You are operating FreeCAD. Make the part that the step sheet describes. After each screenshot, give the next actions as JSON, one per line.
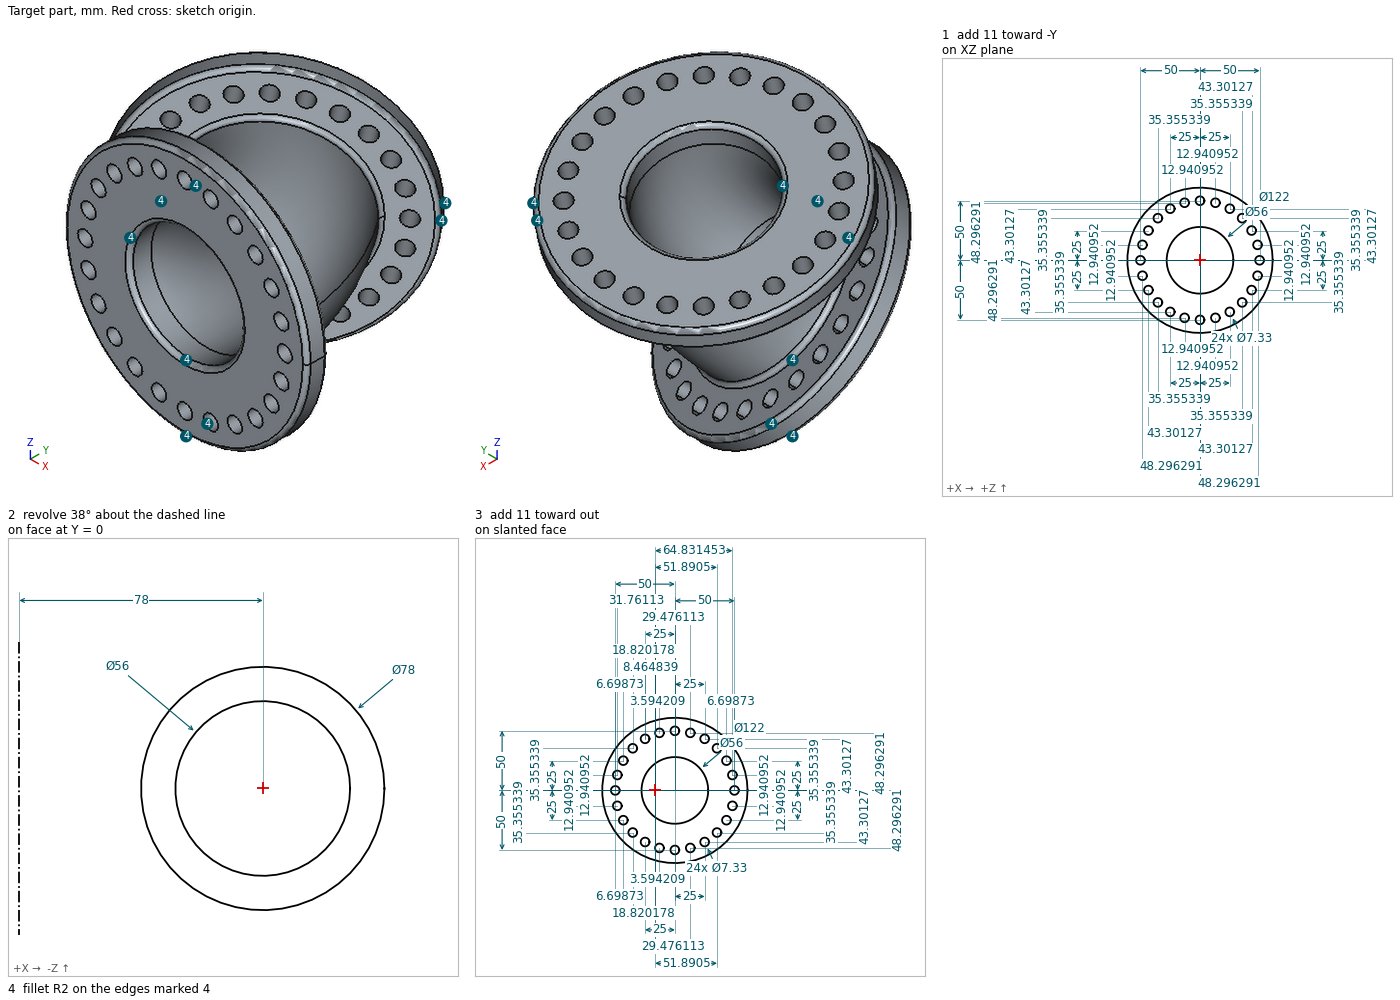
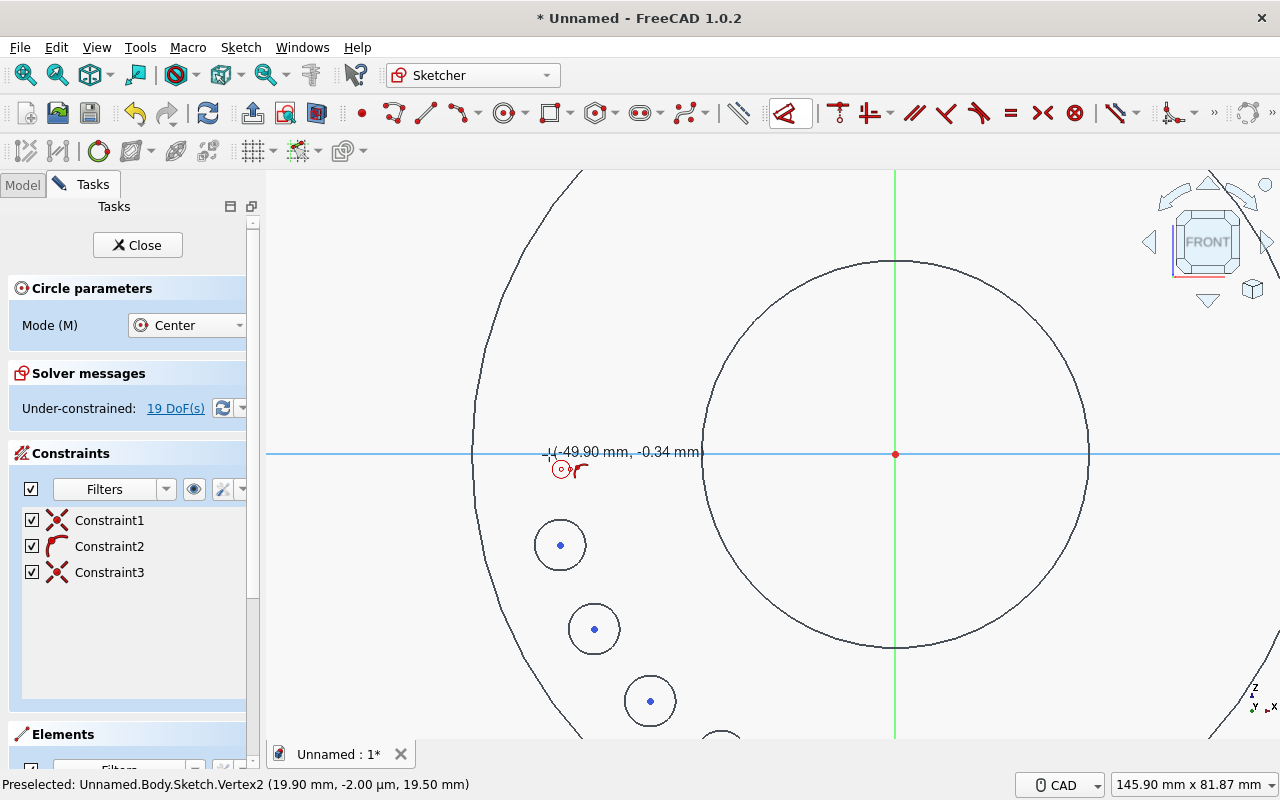
{"action": "left_click", "coordinate": [548, 454]}
{"action": "left_click", "coordinate": [566, 436]}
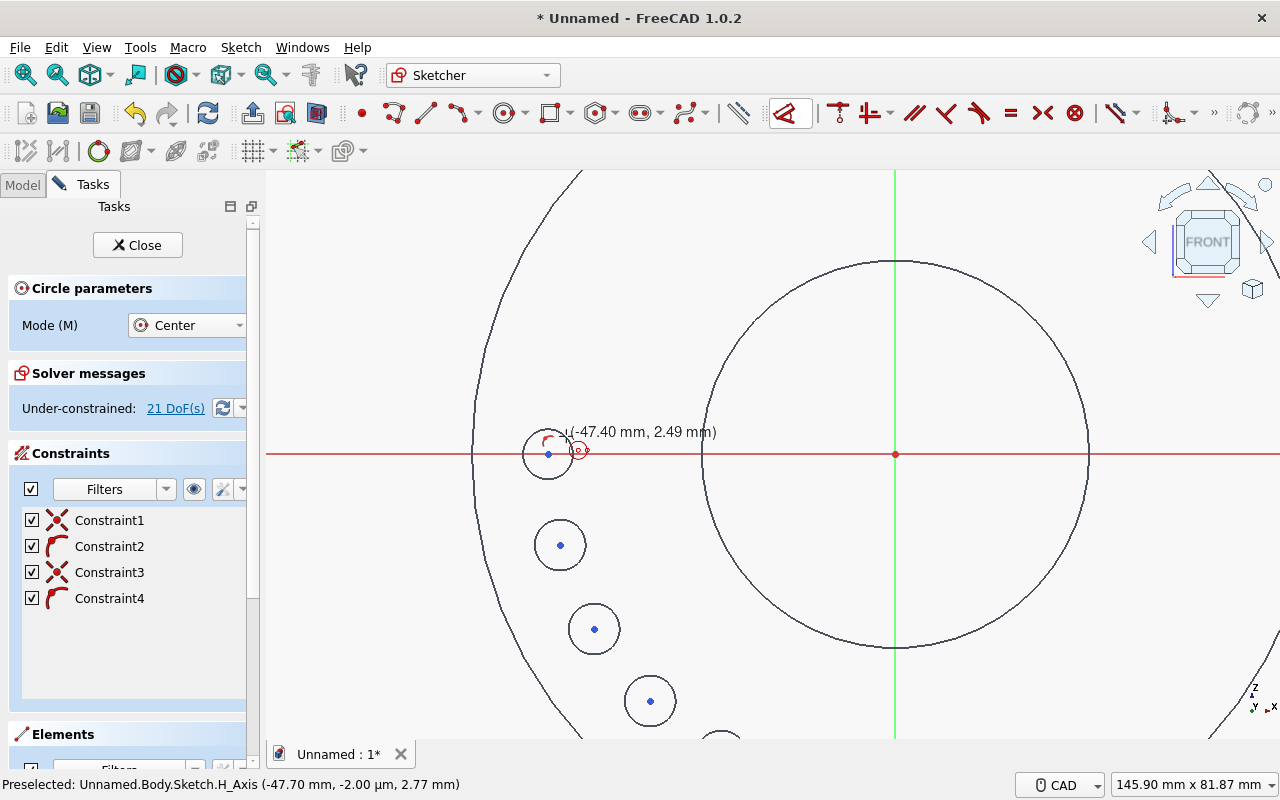
{"action": "left_click", "coordinate": [560, 364]}
{"action": "left_click", "coordinate": [578, 346]}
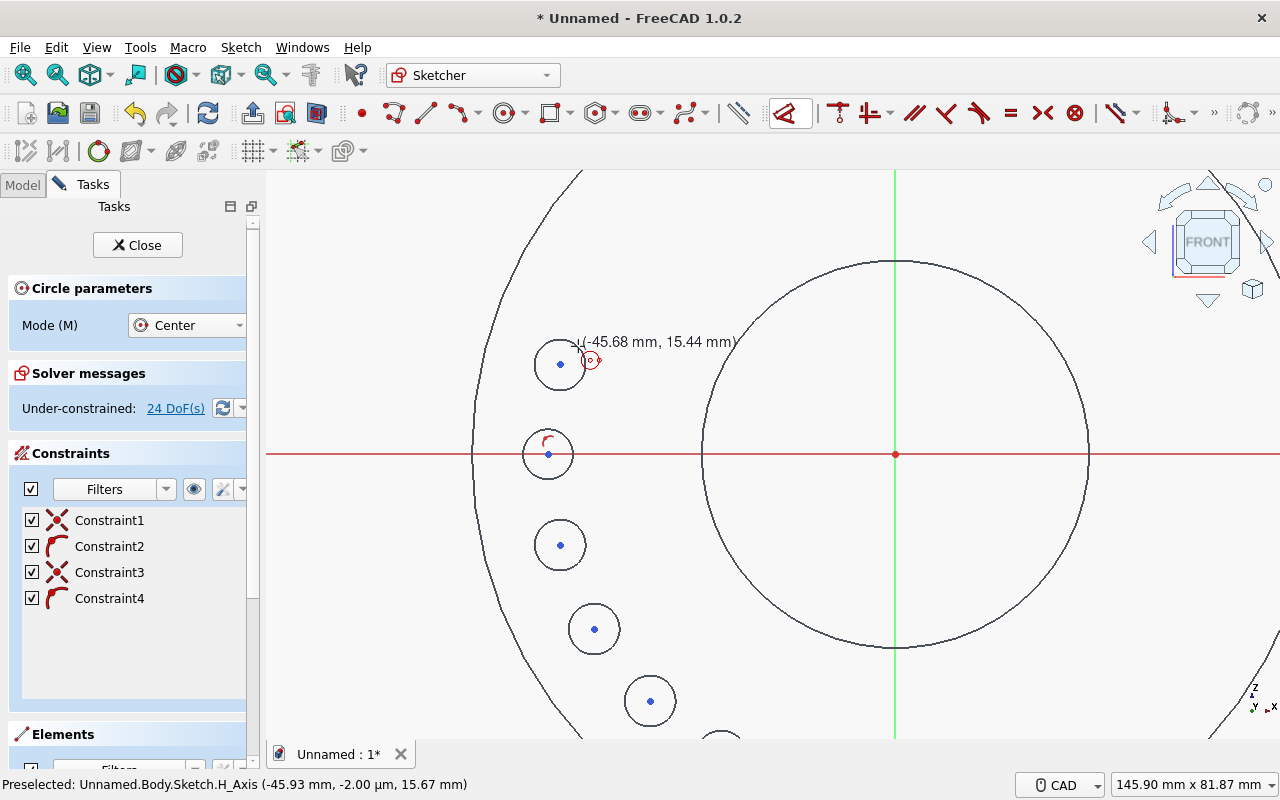
{"action": "left_click", "coordinate": [595, 281]}
{"action": "left_click", "coordinate": [613, 263]}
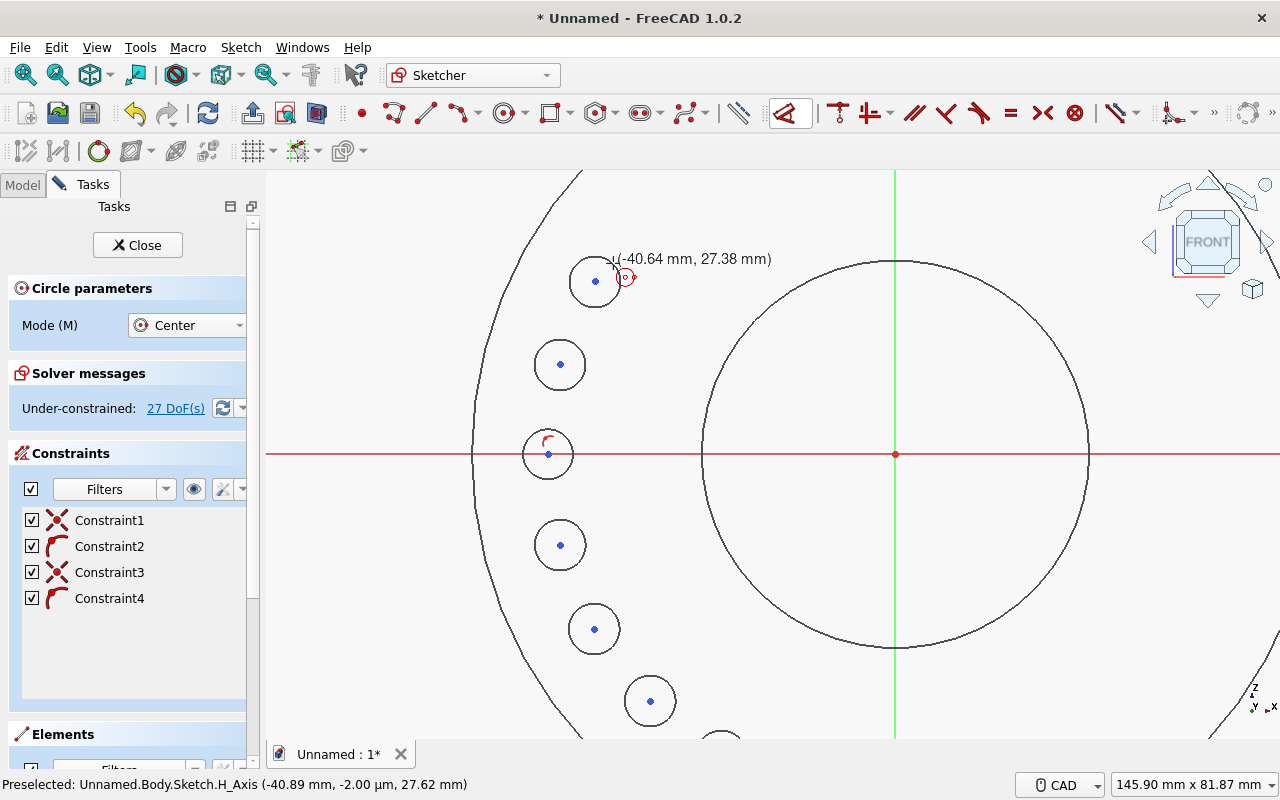
{"action": "left_click", "coordinate": [650, 209]}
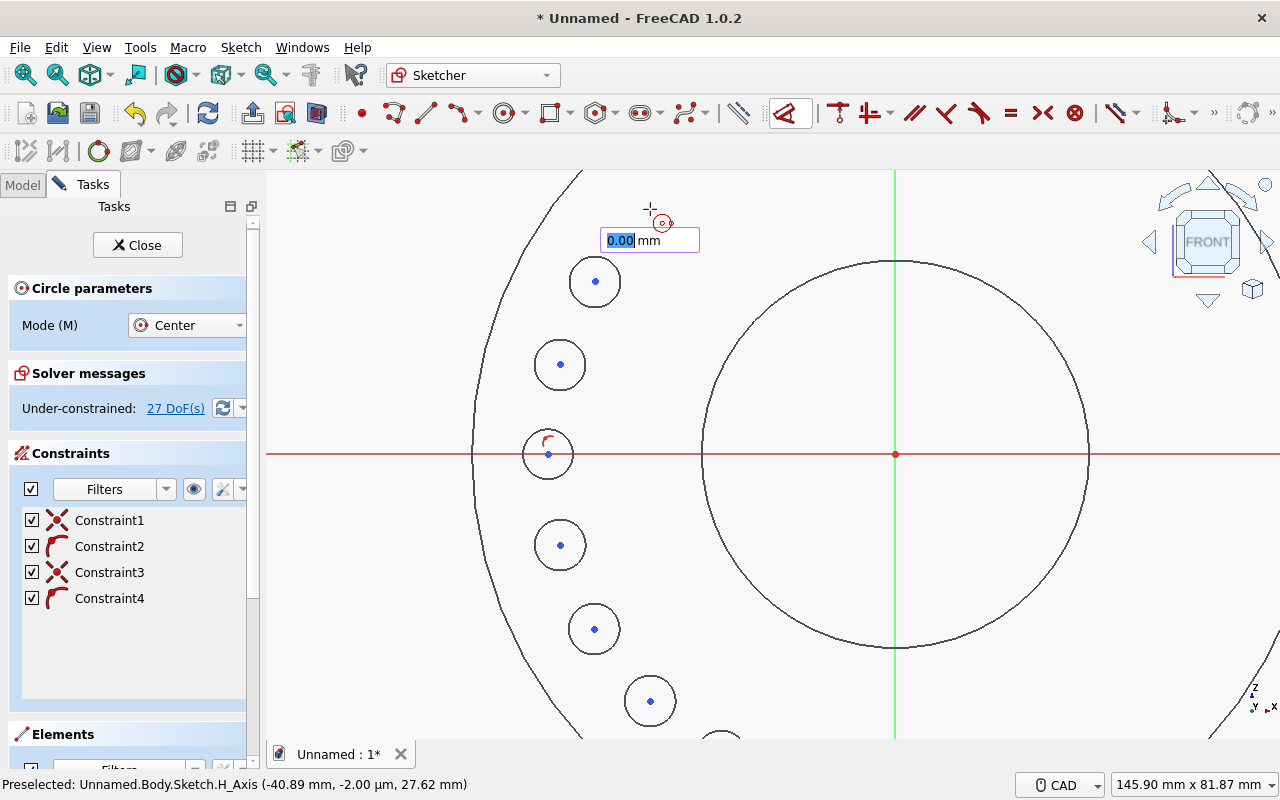
{"action": "scroll", "coordinate": [549, 455], "scroll_direction": "down", "scroll_amount": 4}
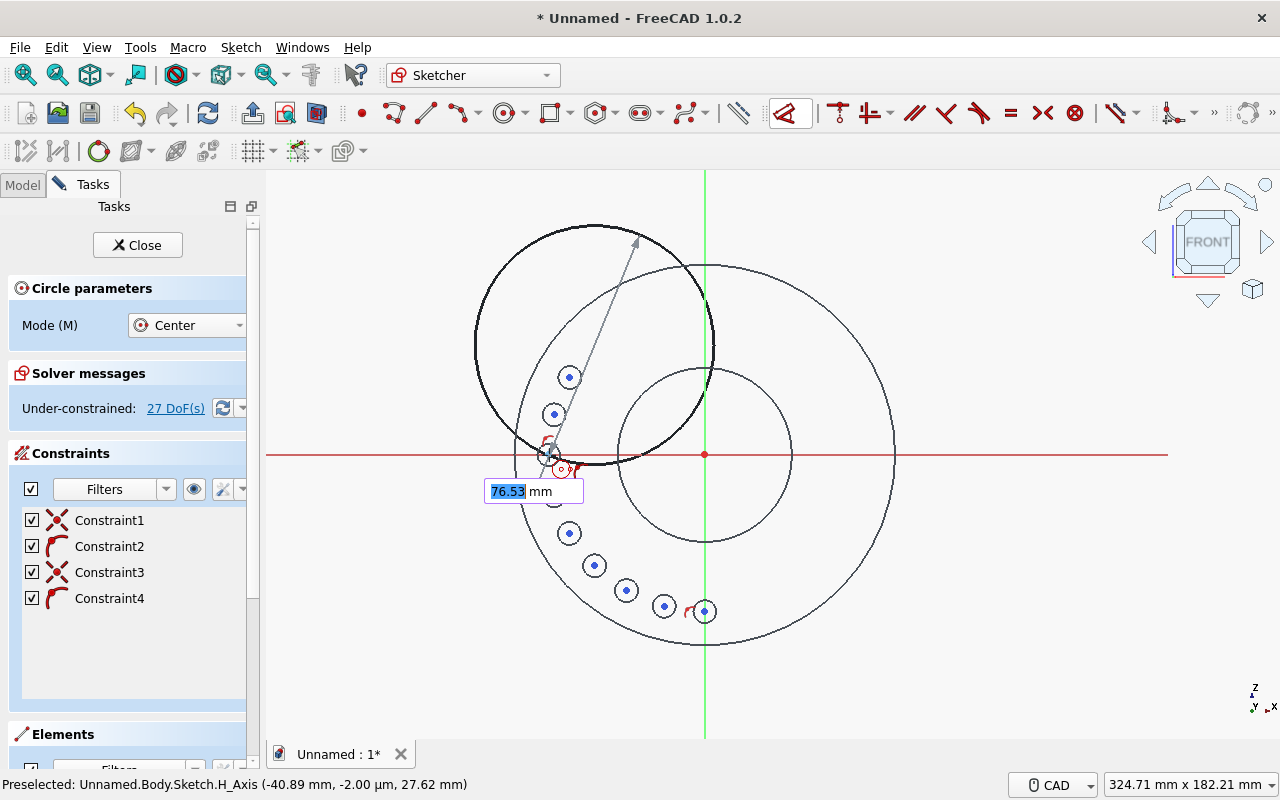
{"action": "scroll", "coordinate": [603, 336], "scroll_direction": "up", "scroll_amount": 2}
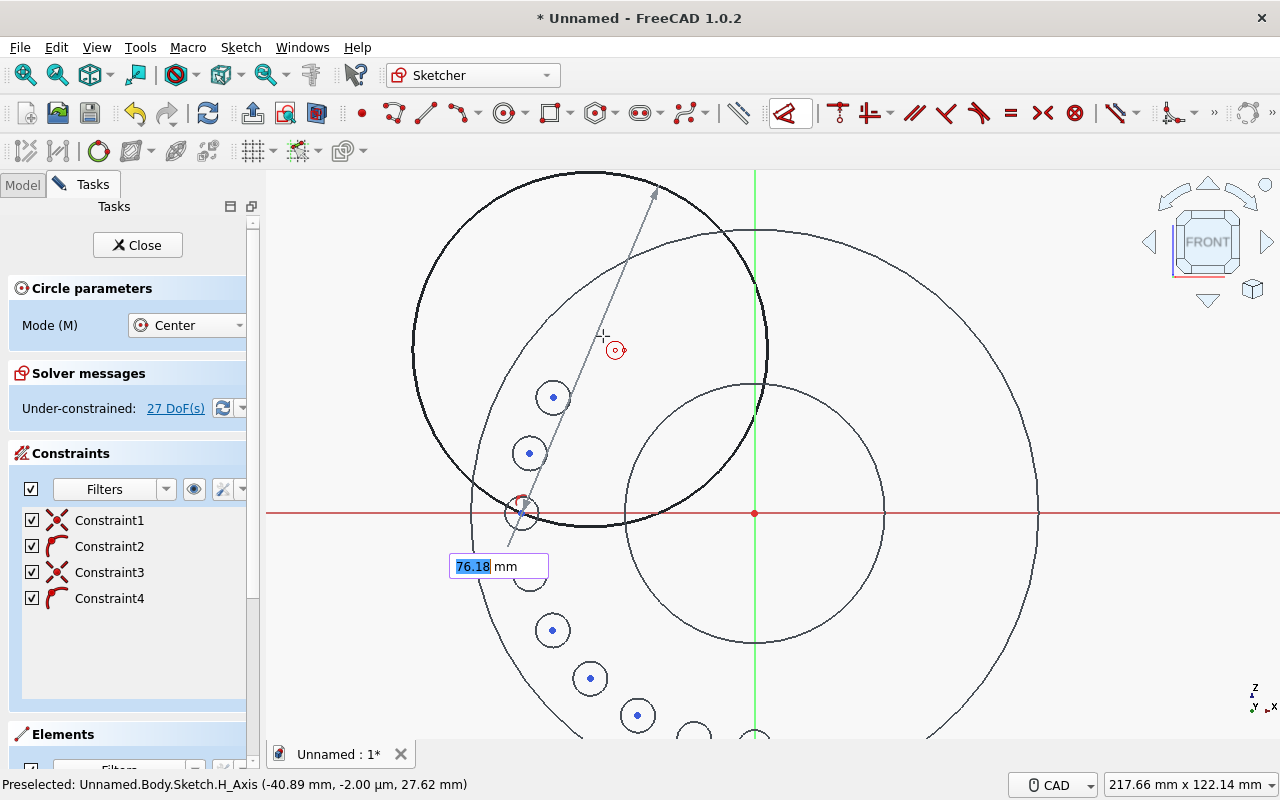
{"action": "left_click", "coordinate": [602, 337]}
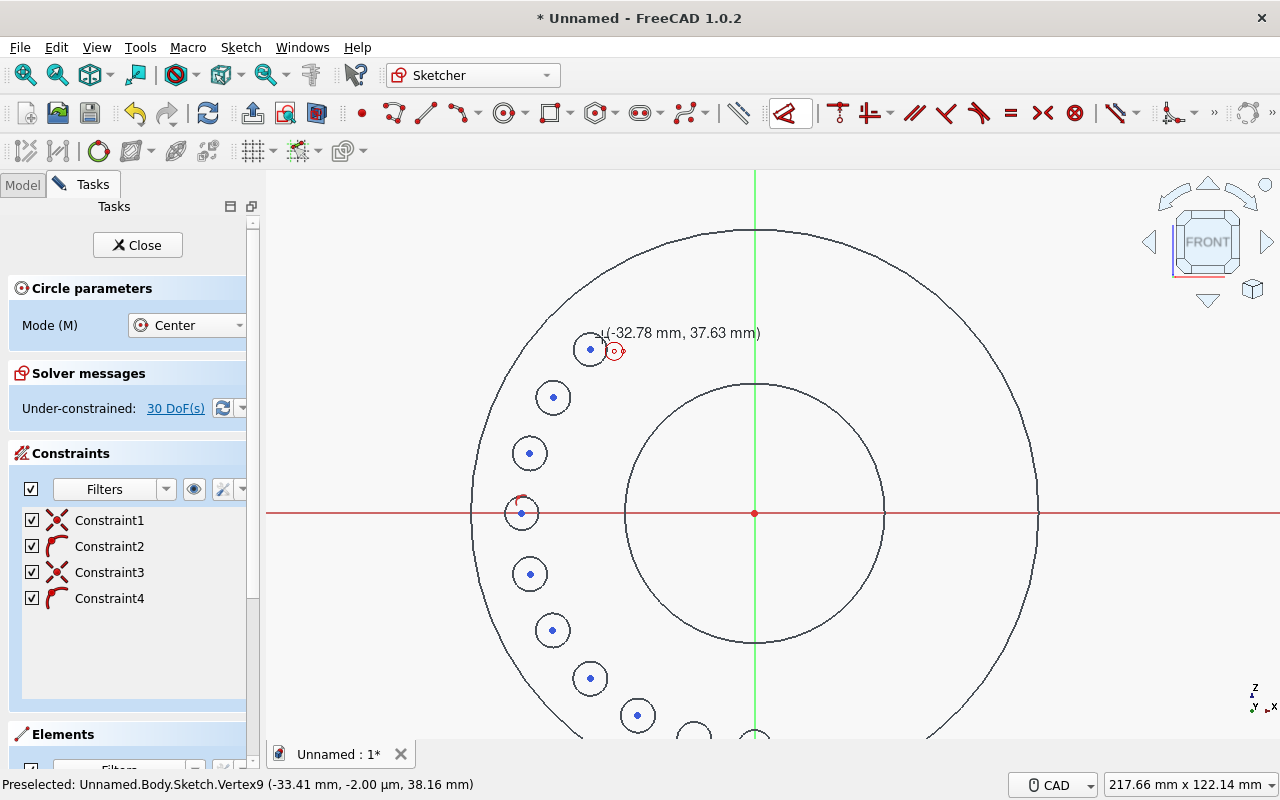
{"action": "scroll", "coordinate": [638, 312], "scroll_direction": "up", "scroll_amount": 2}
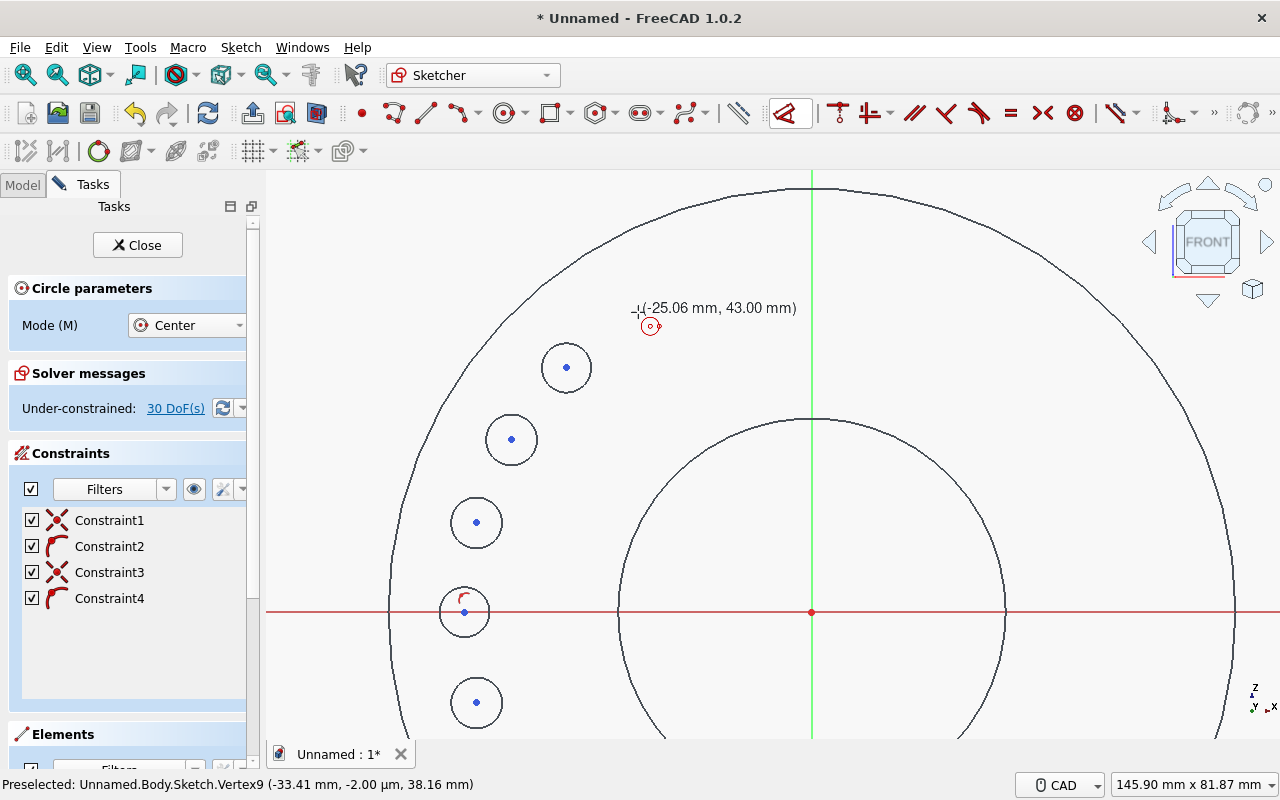
{"action": "left_click", "coordinate": [638, 311]}
{"action": "left_click", "coordinate": [656, 293]}